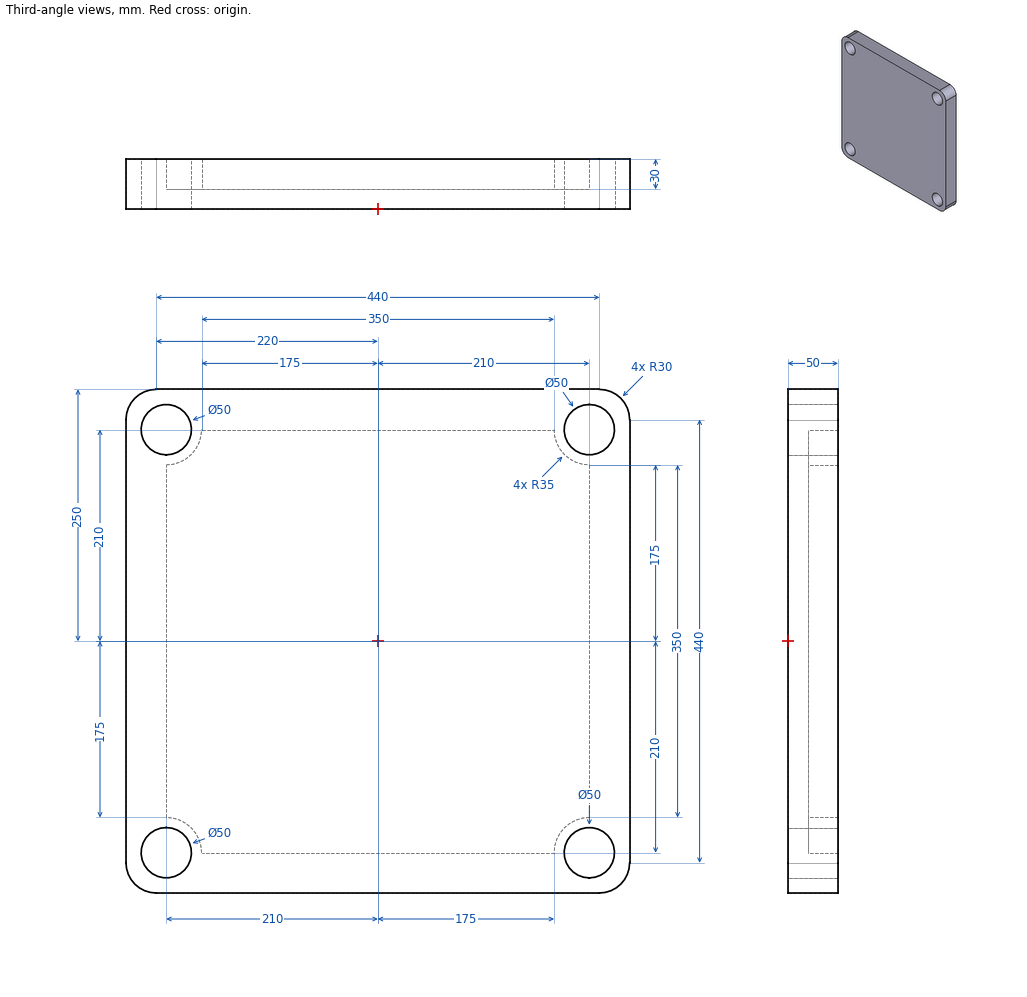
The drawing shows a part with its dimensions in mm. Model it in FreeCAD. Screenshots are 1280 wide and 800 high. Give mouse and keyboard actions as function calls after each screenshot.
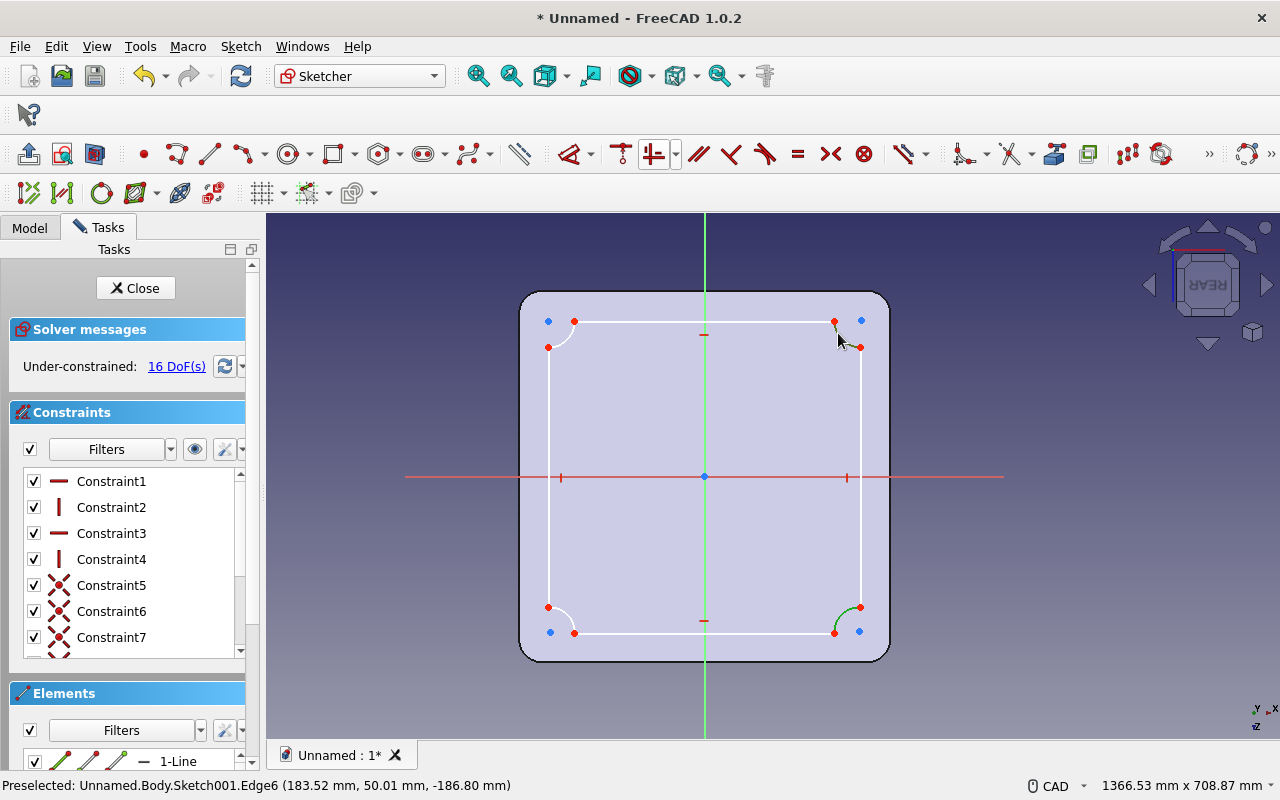
click(560, 345)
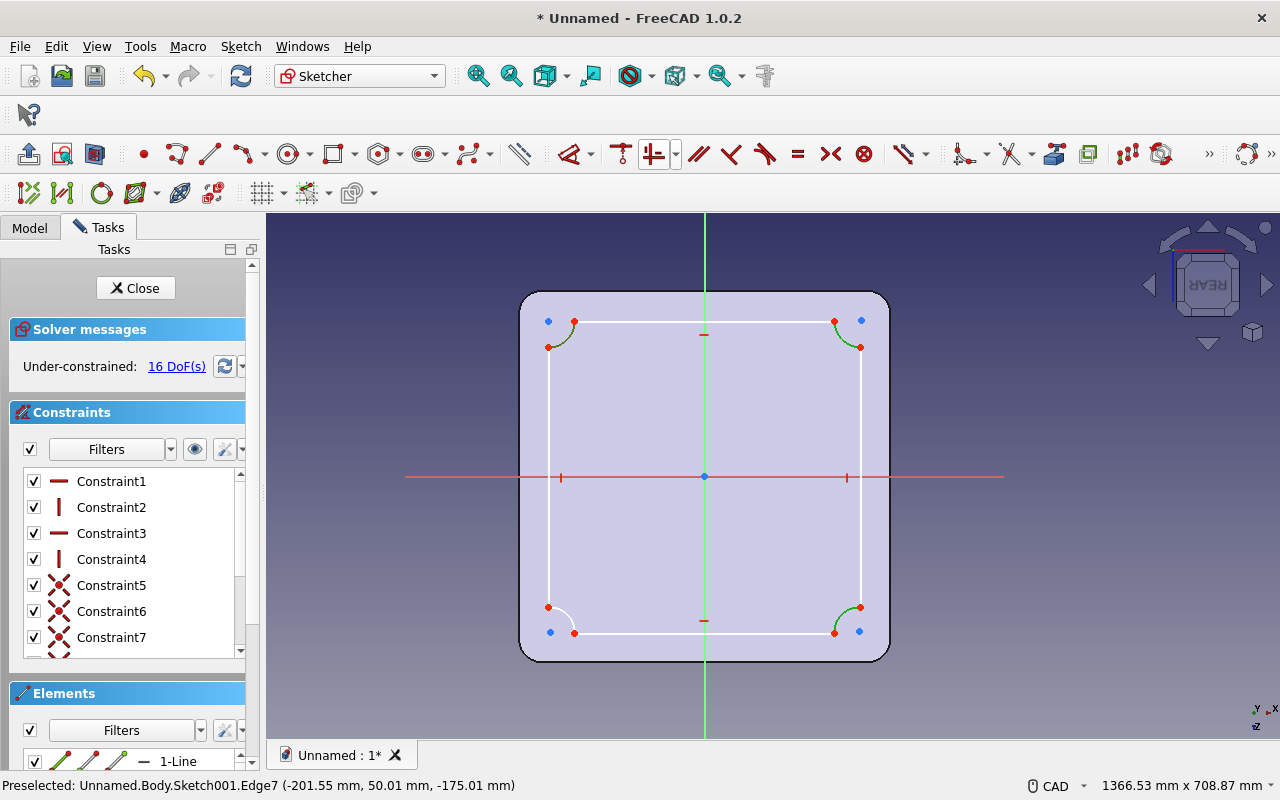
click(572, 621)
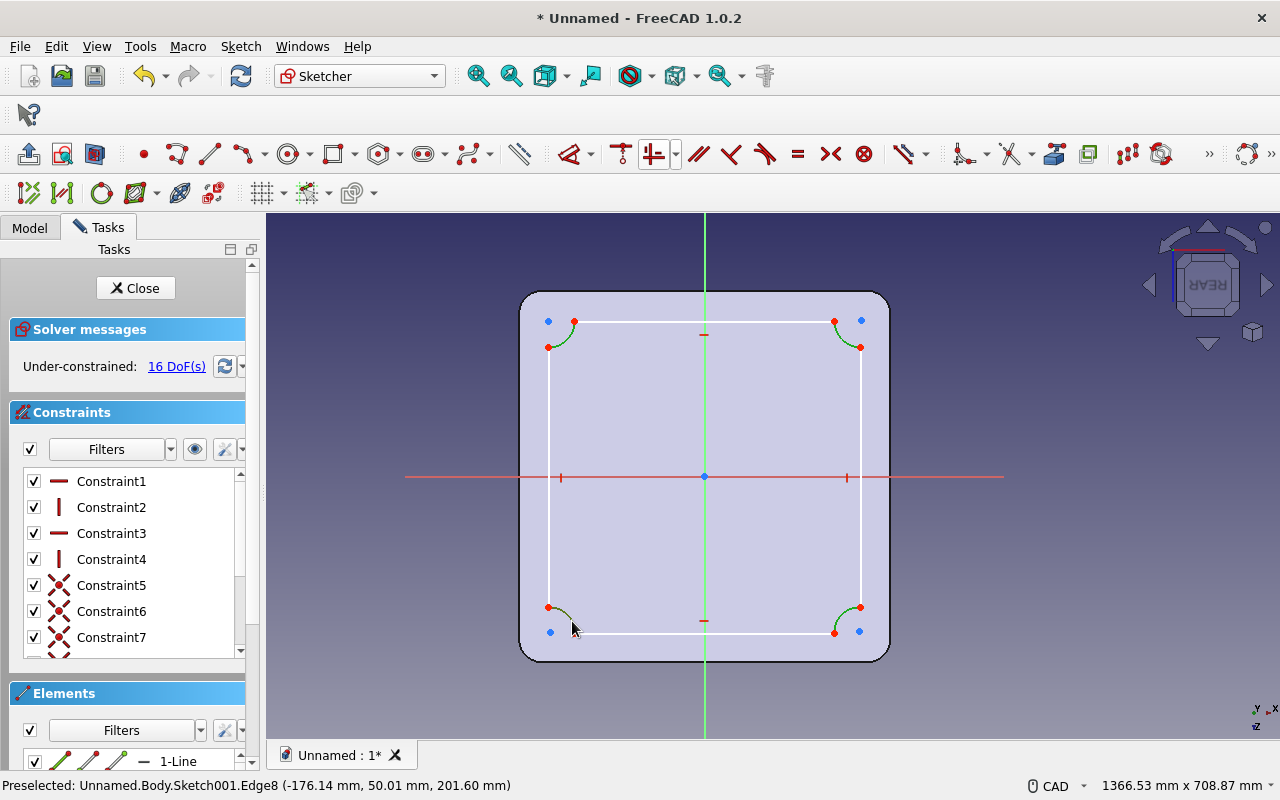
click(798, 154)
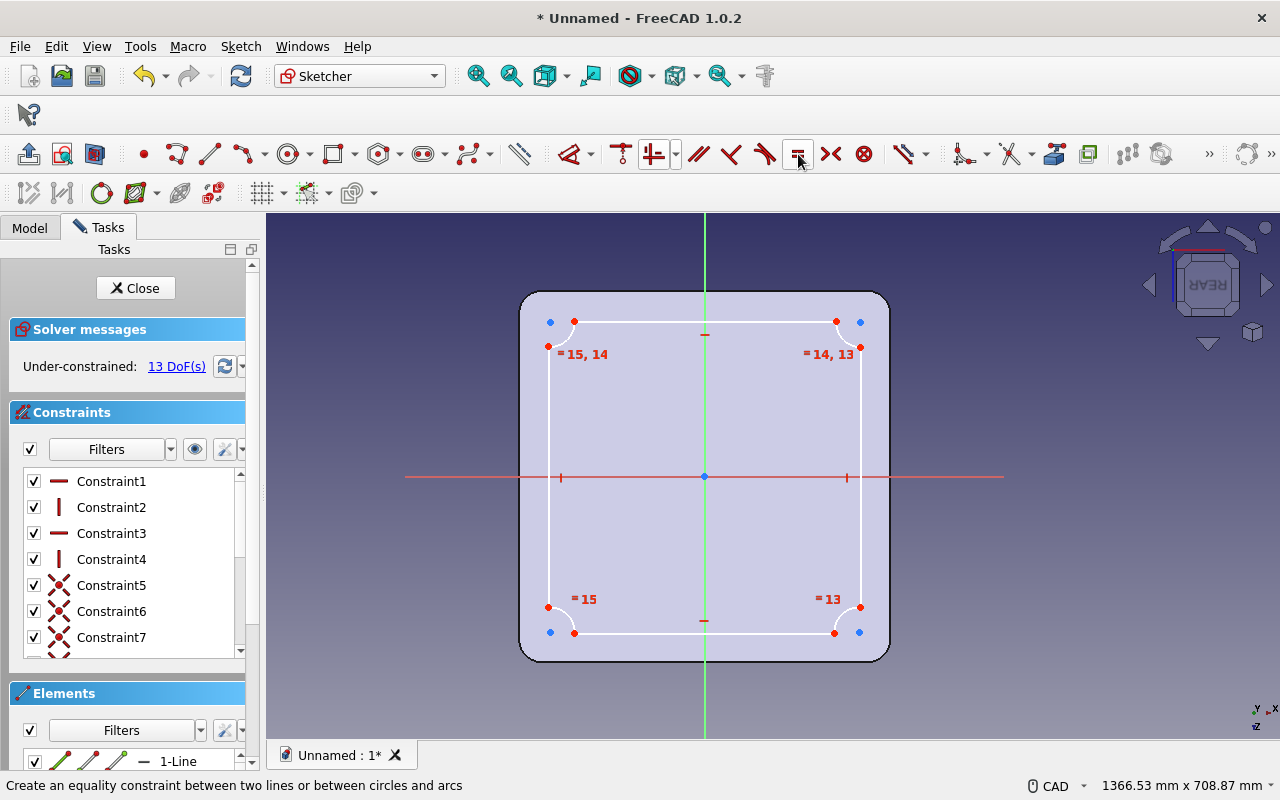
click(568, 154)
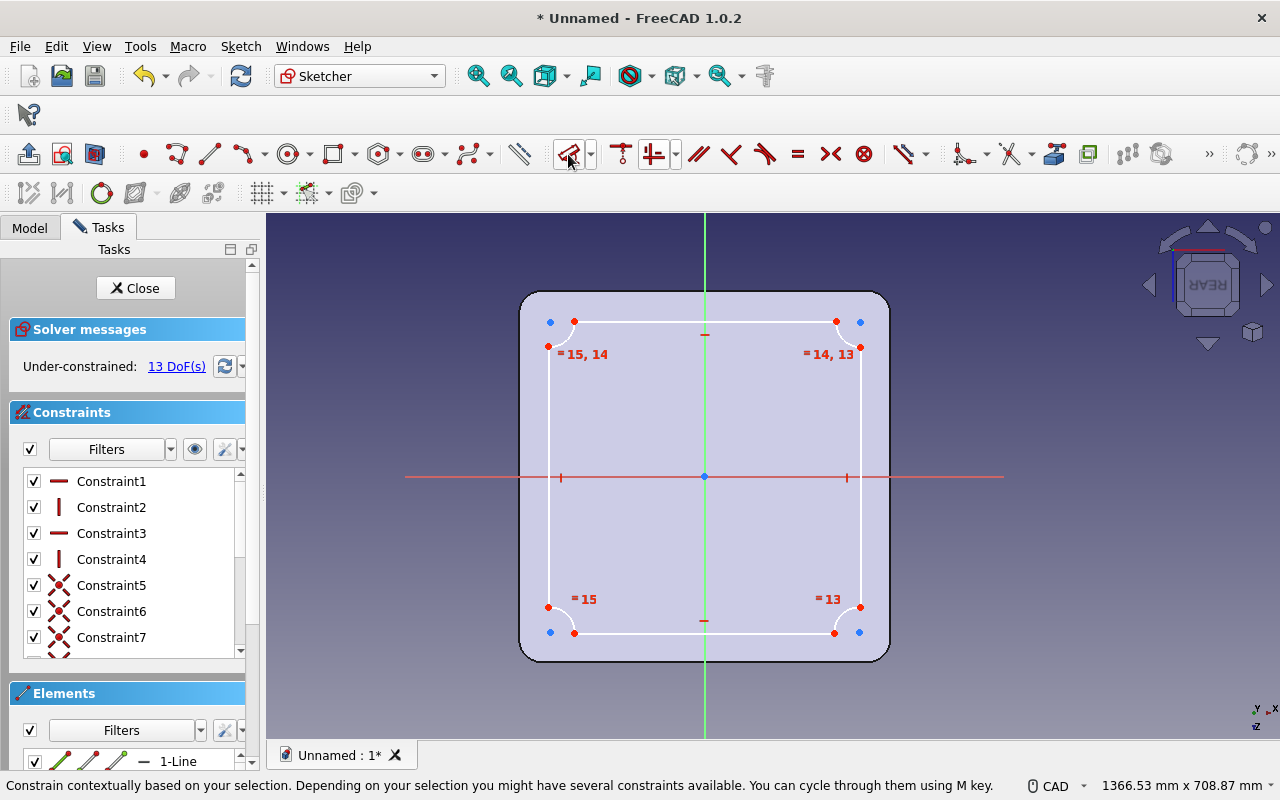
scroll(849, 610, up, 3)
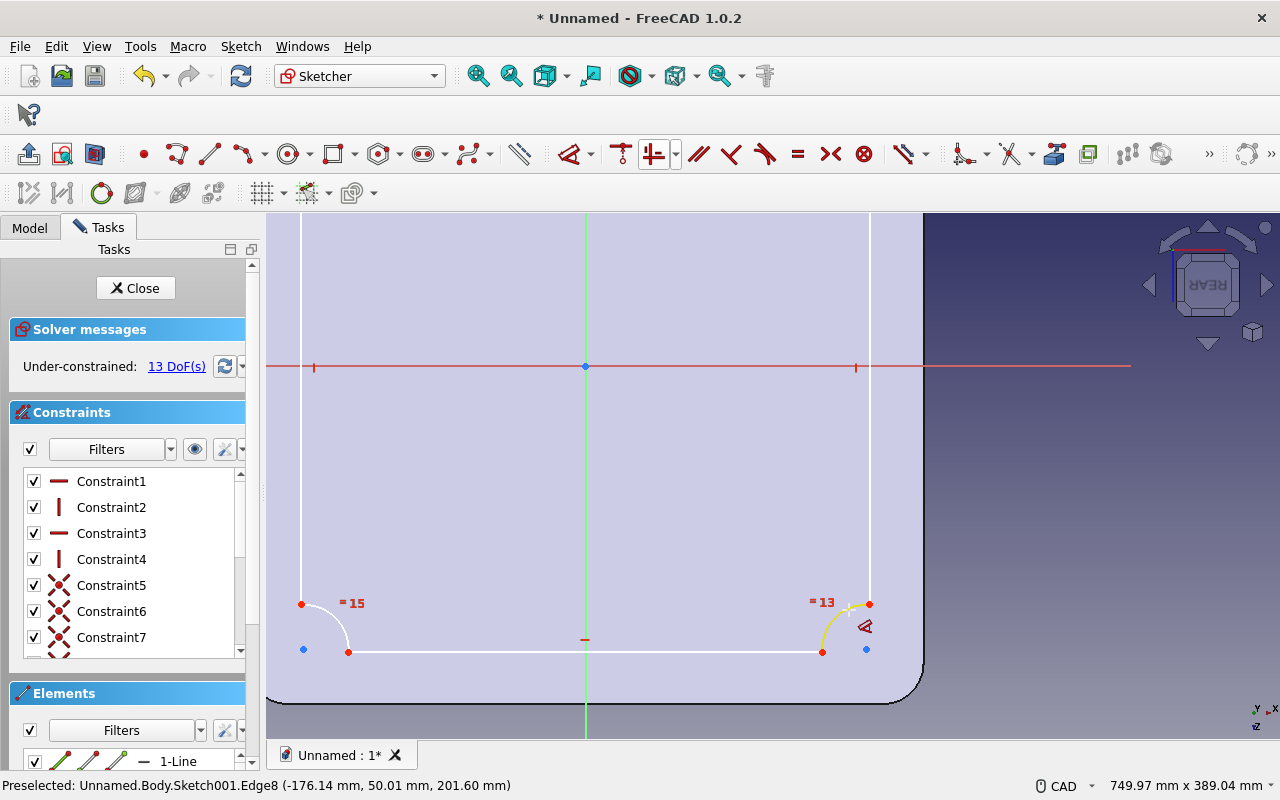
click(848, 609)
click(834, 580)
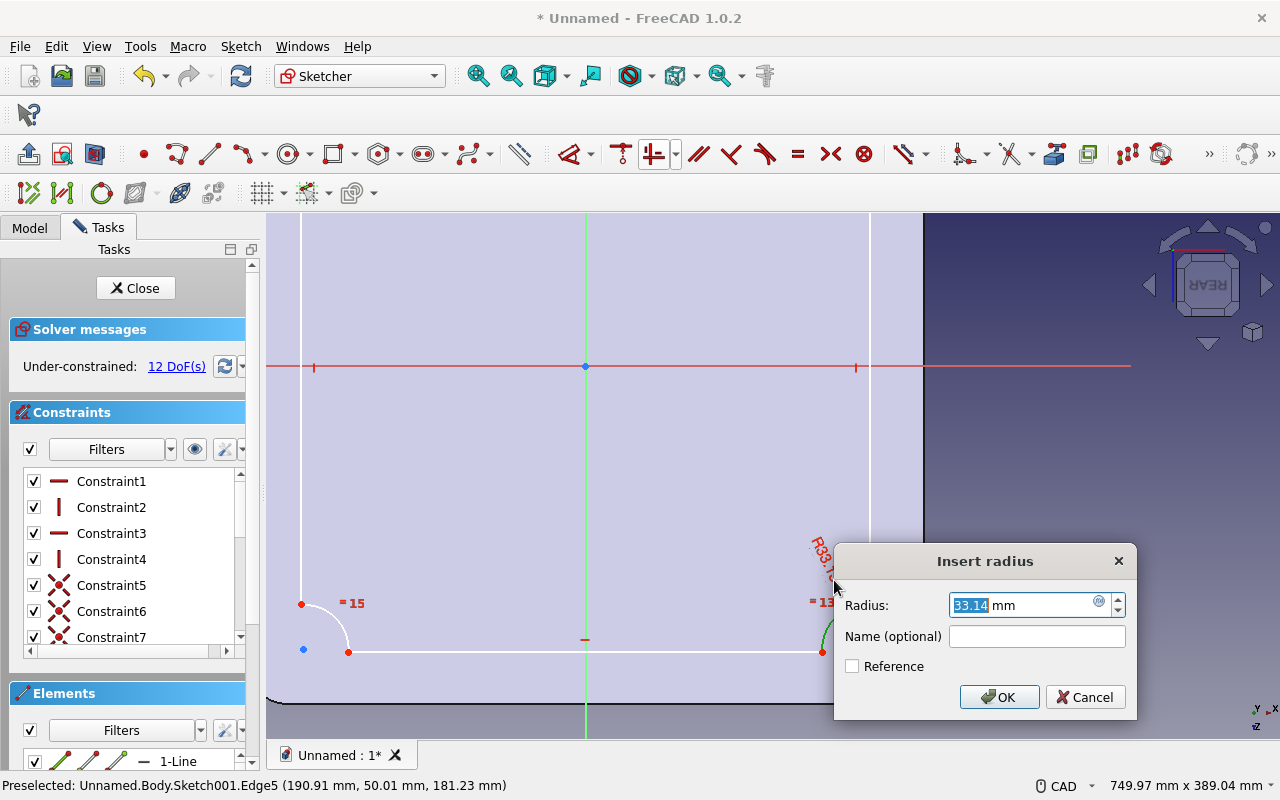
text(35)
key(Return)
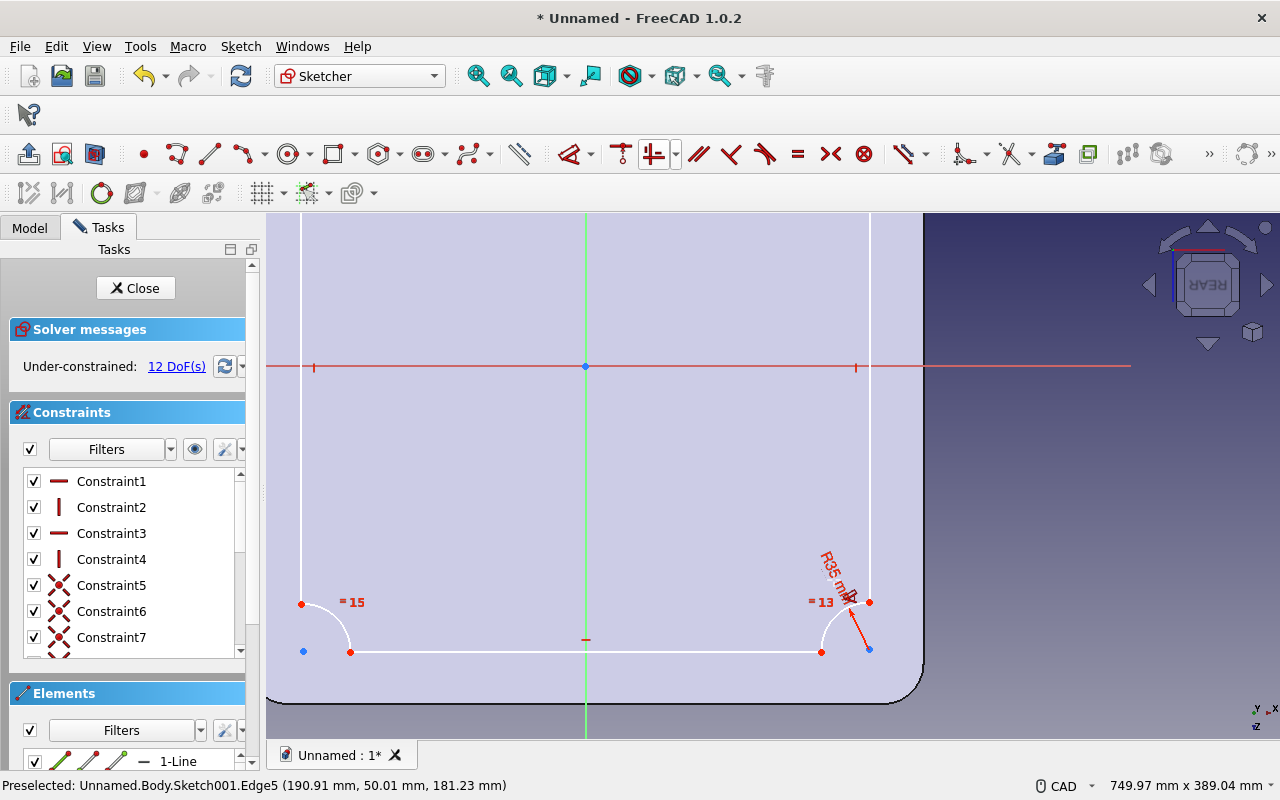
click(492, 652)
click(478, 686)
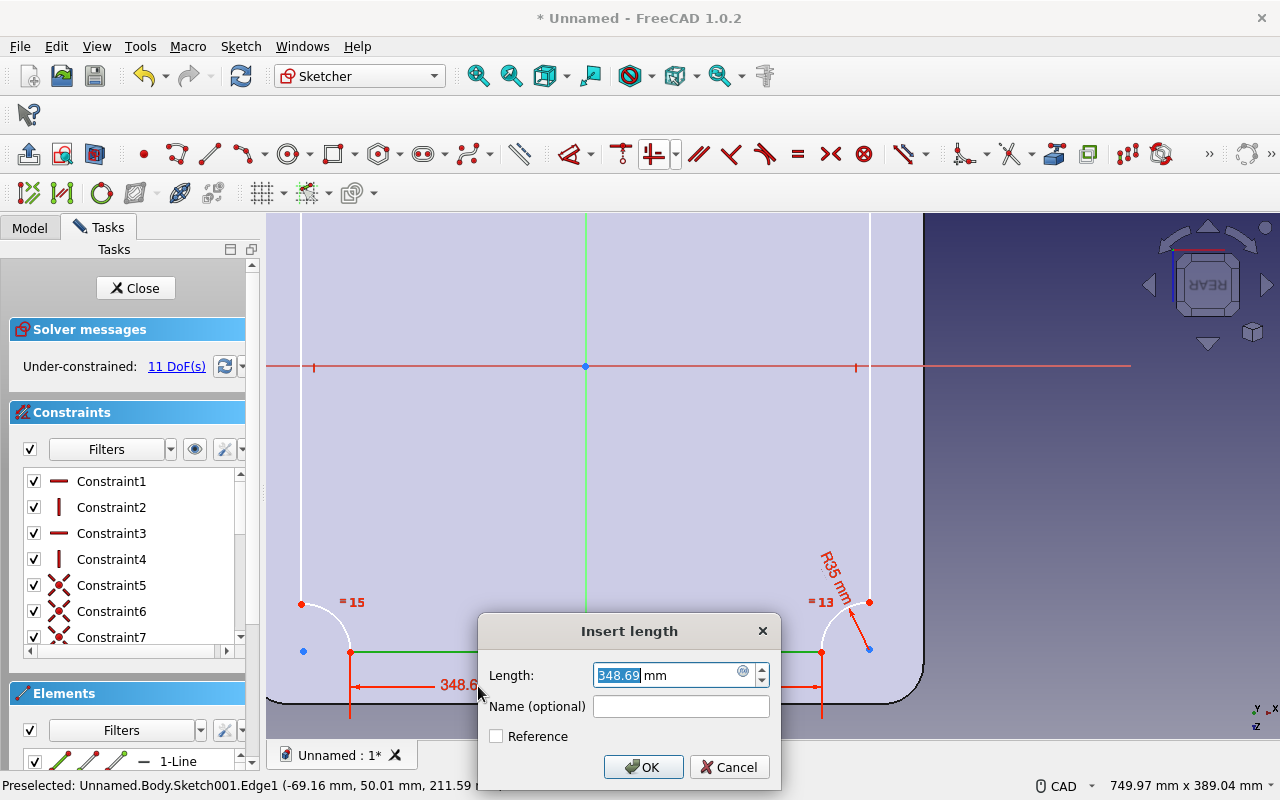
text(350)
key(Return)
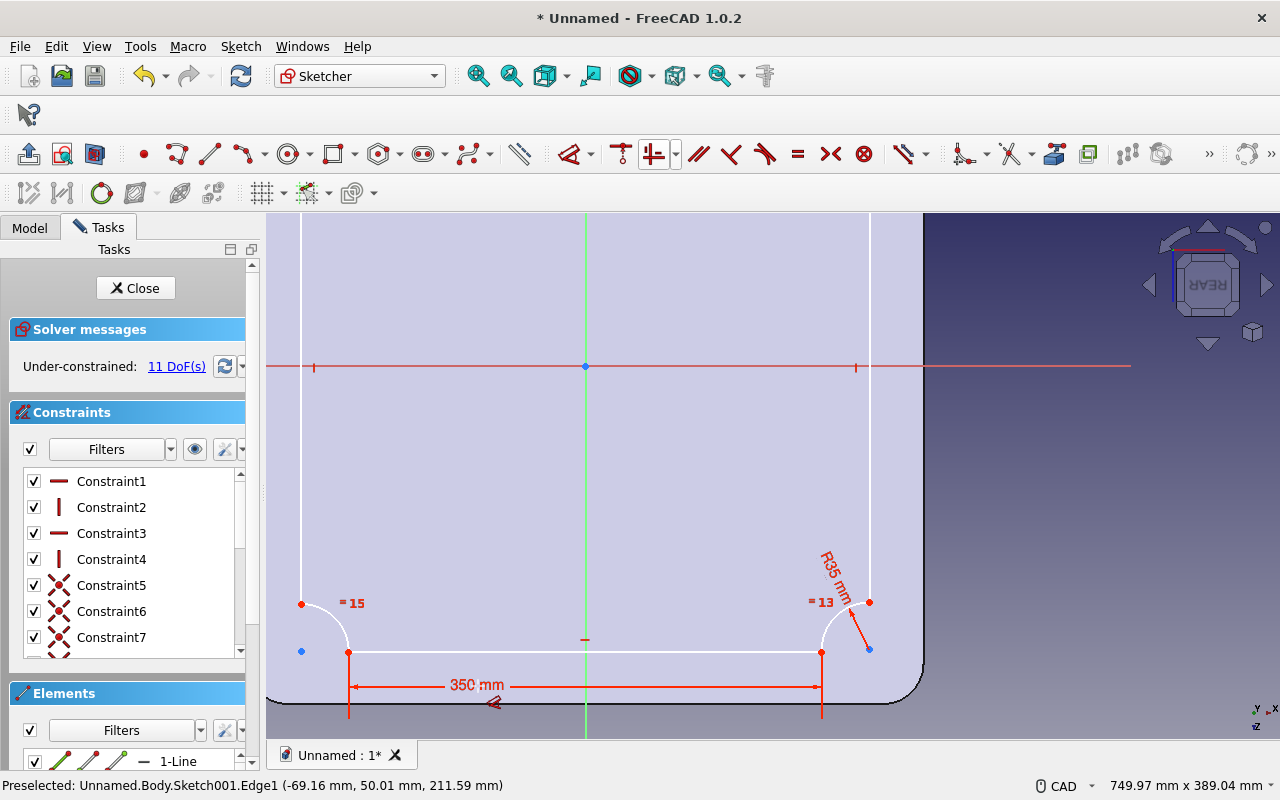
click(870, 462)
click(904, 422)